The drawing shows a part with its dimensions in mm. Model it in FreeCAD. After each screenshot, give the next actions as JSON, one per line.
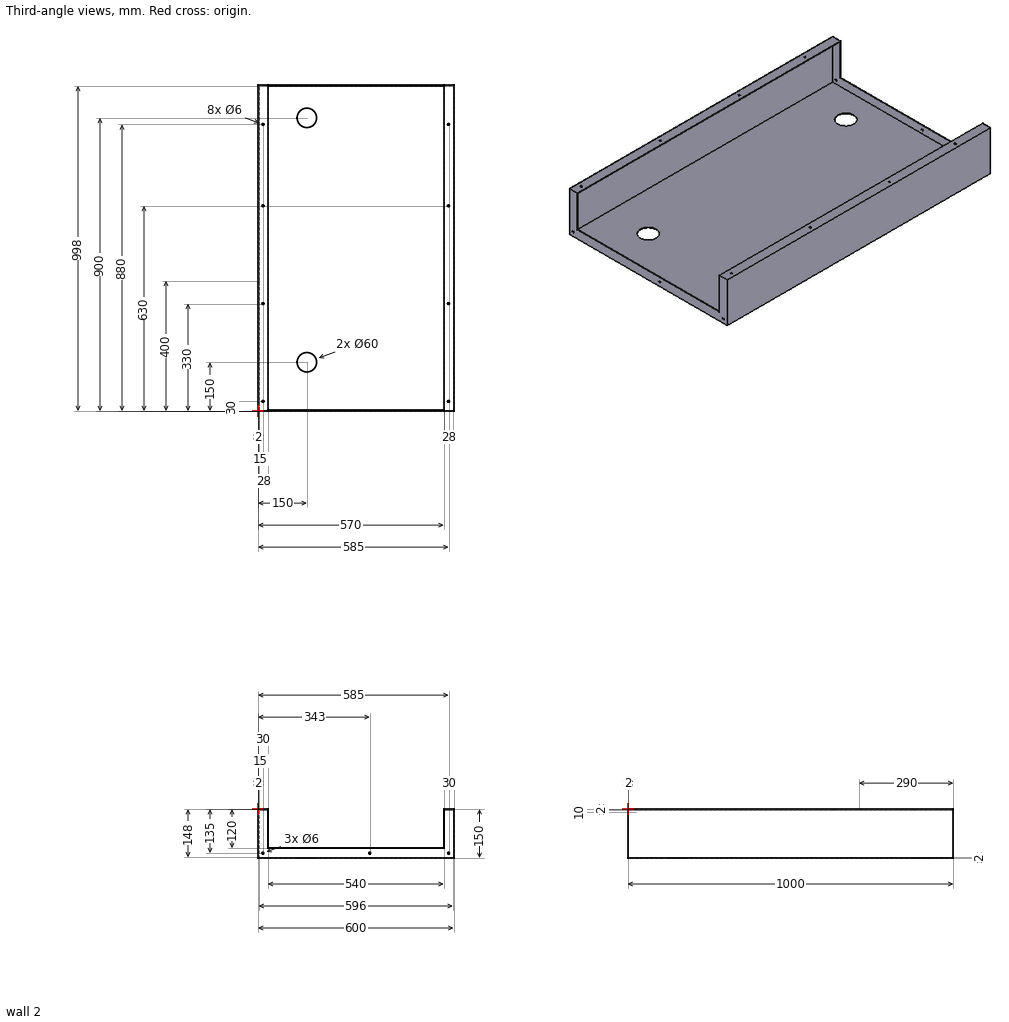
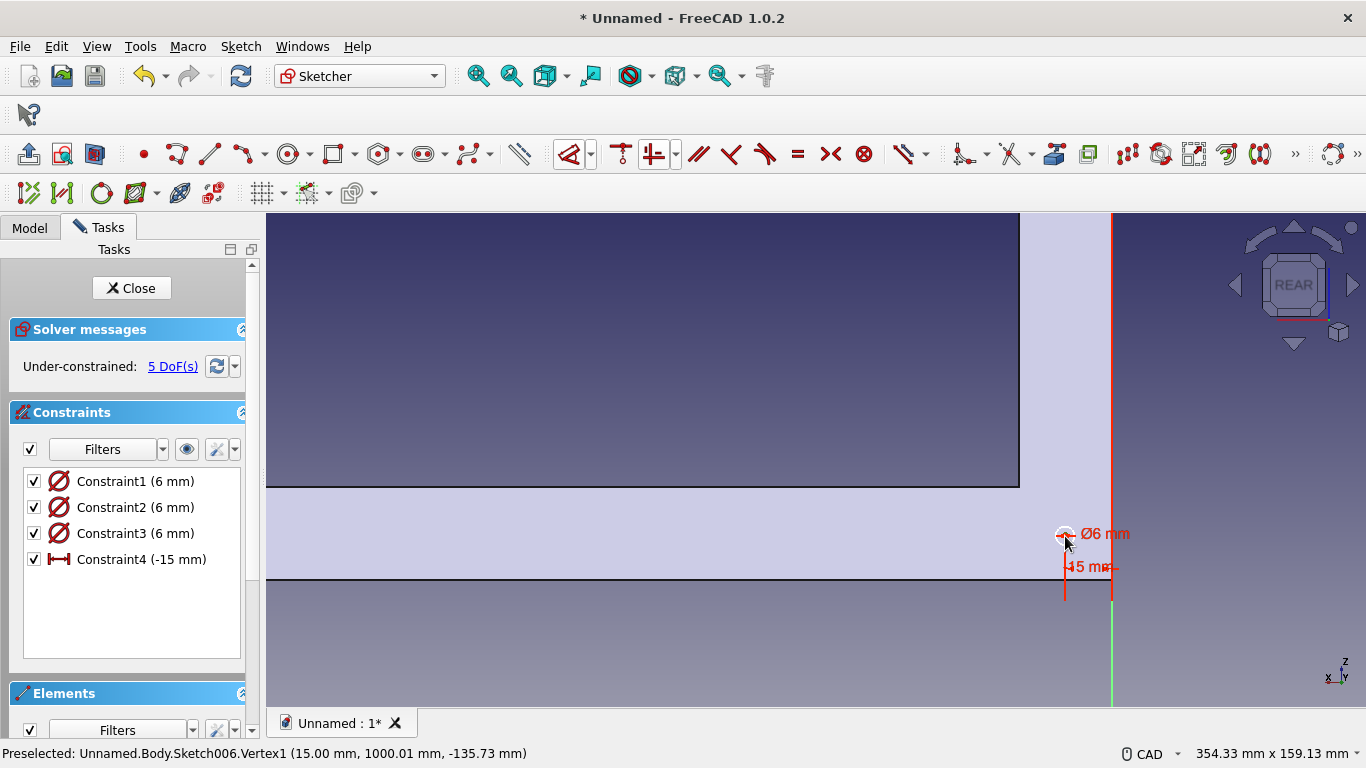
{"action": "left_click", "coordinate": [590, 154]}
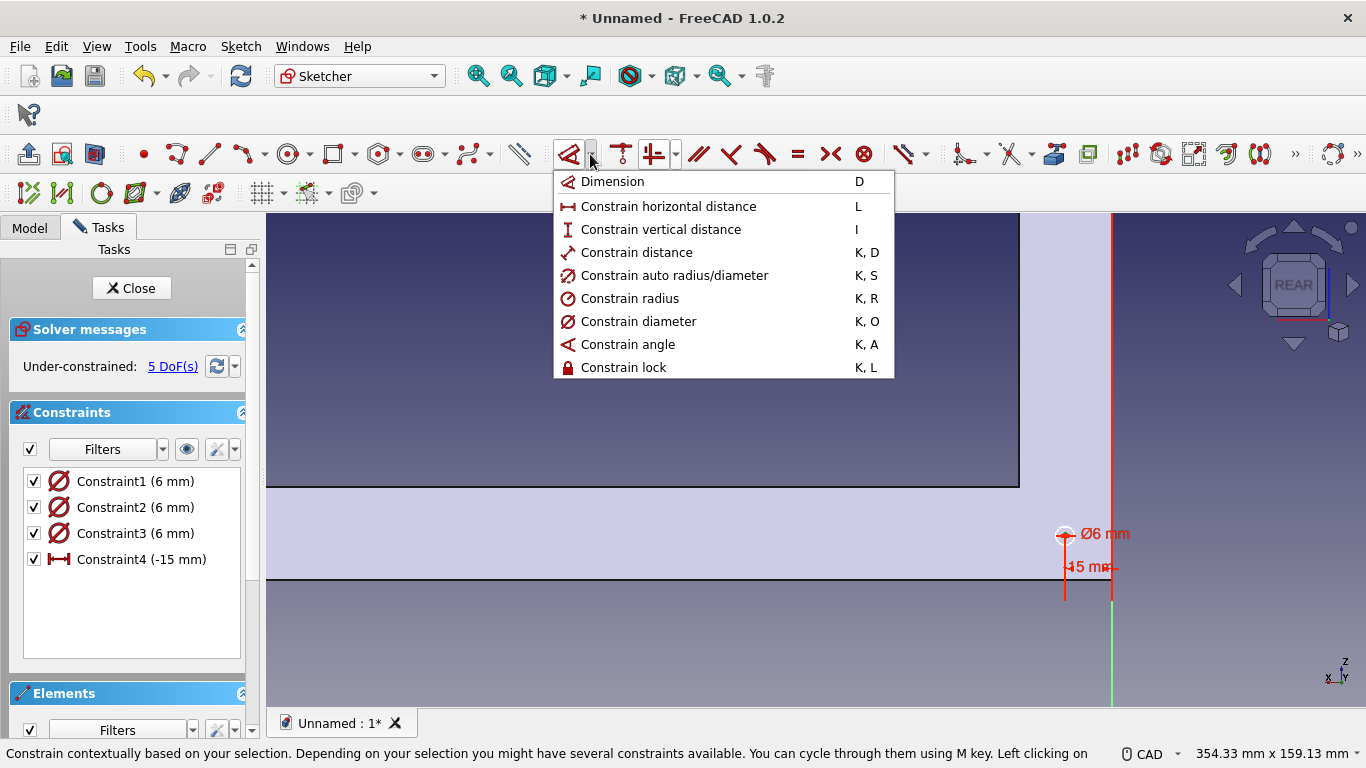
{"action": "left_click", "coordinate": [724, 230]}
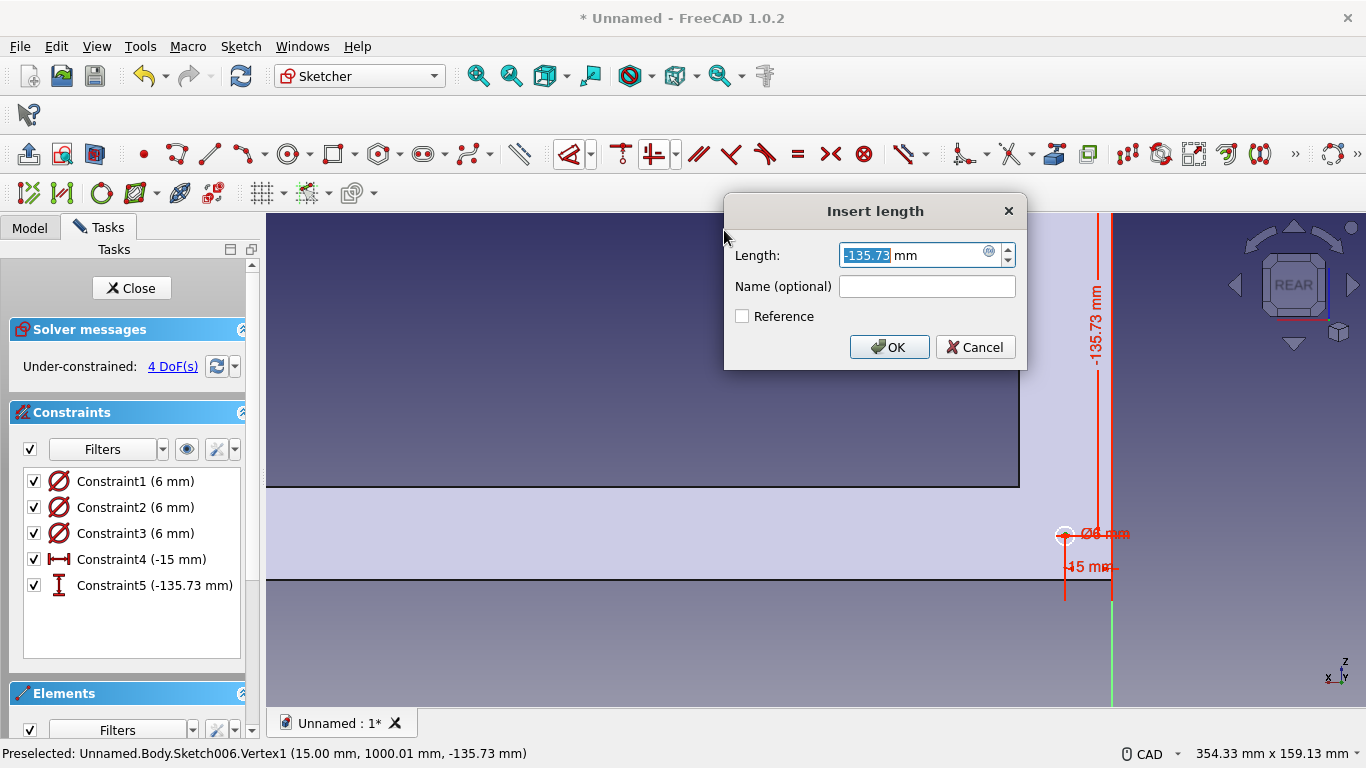
{"action": "type", "text": "-135"}
{"action": "key", "text": "Return"}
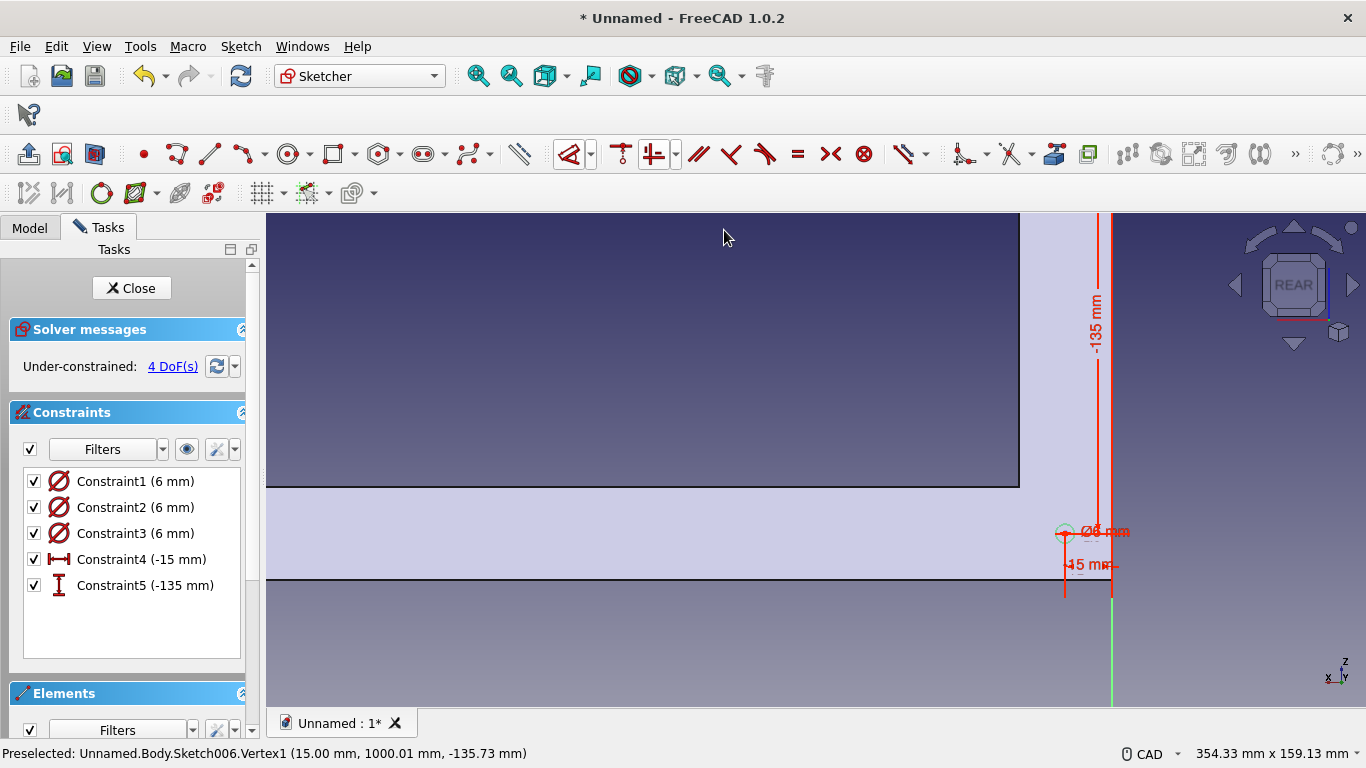
{"action": "scroll", "coordinate": [1067, 536], "scroll_direction": "down", "scroll_amount": 5}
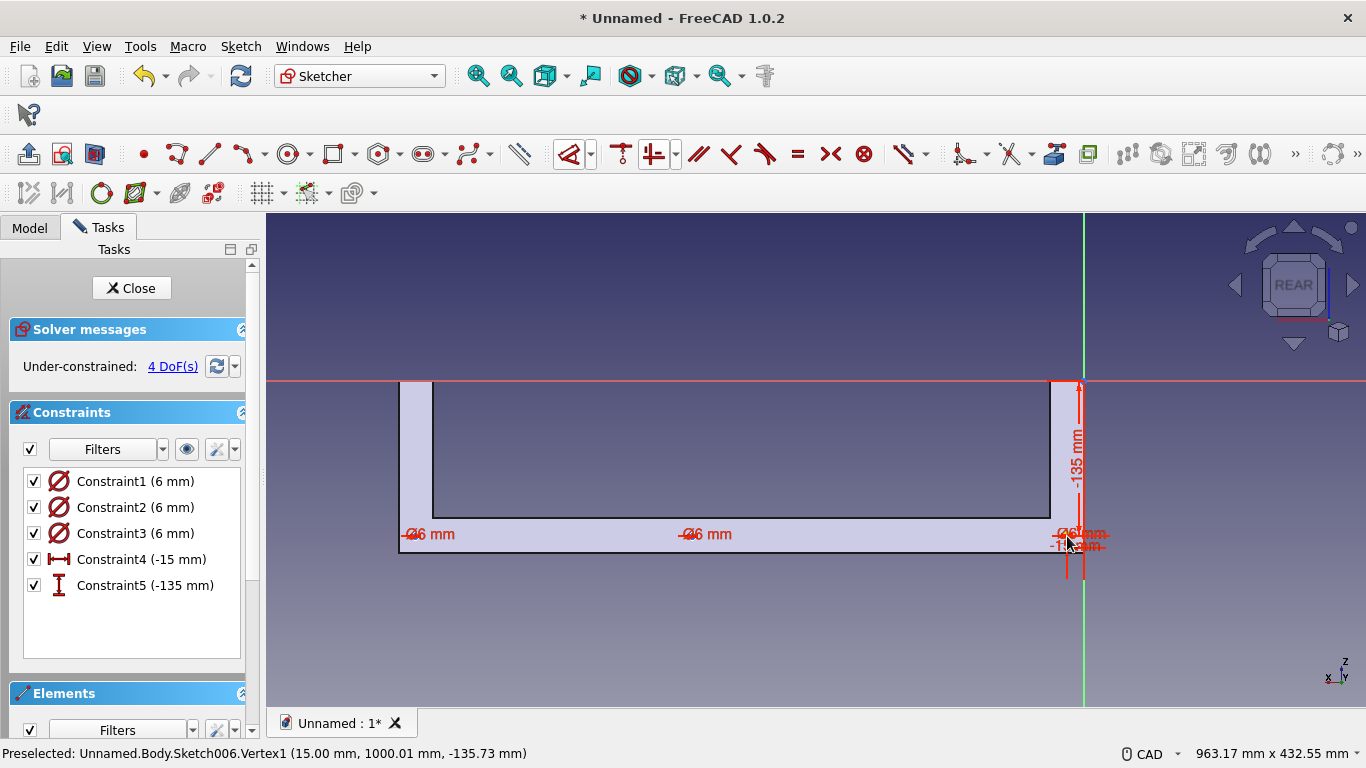
{"action": "left_click", "coordinate": [693, 536]}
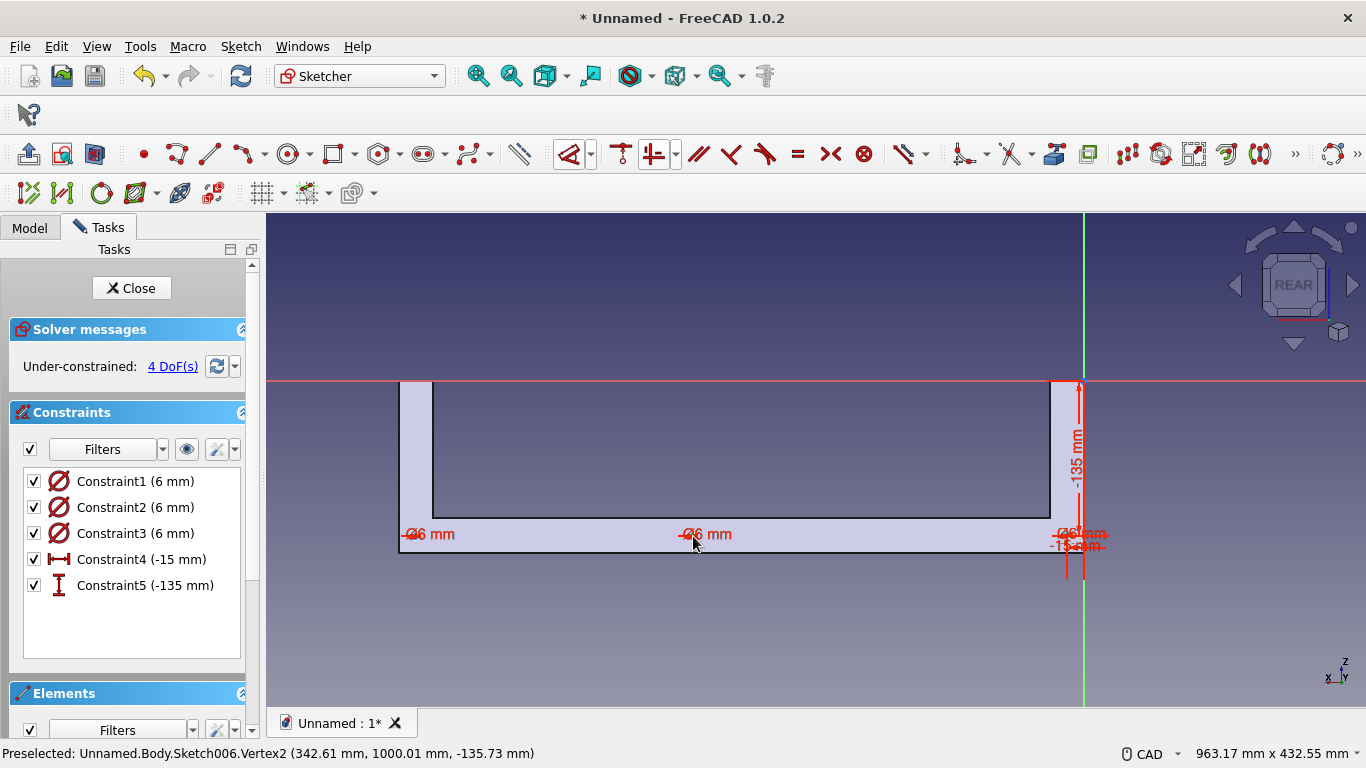
{"action": "left_click", "coordinate": [590, 154]}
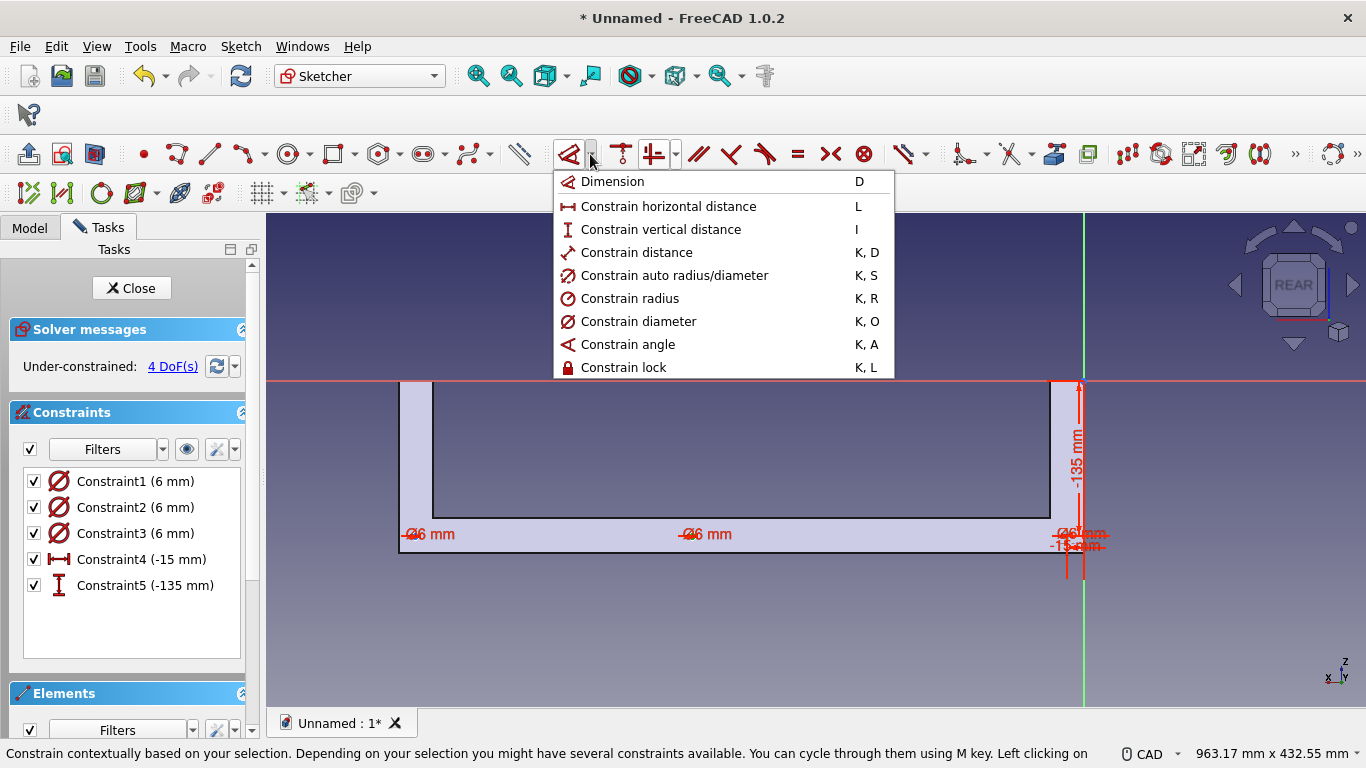
{"action": "left_click", "coordinate": [724, 206]}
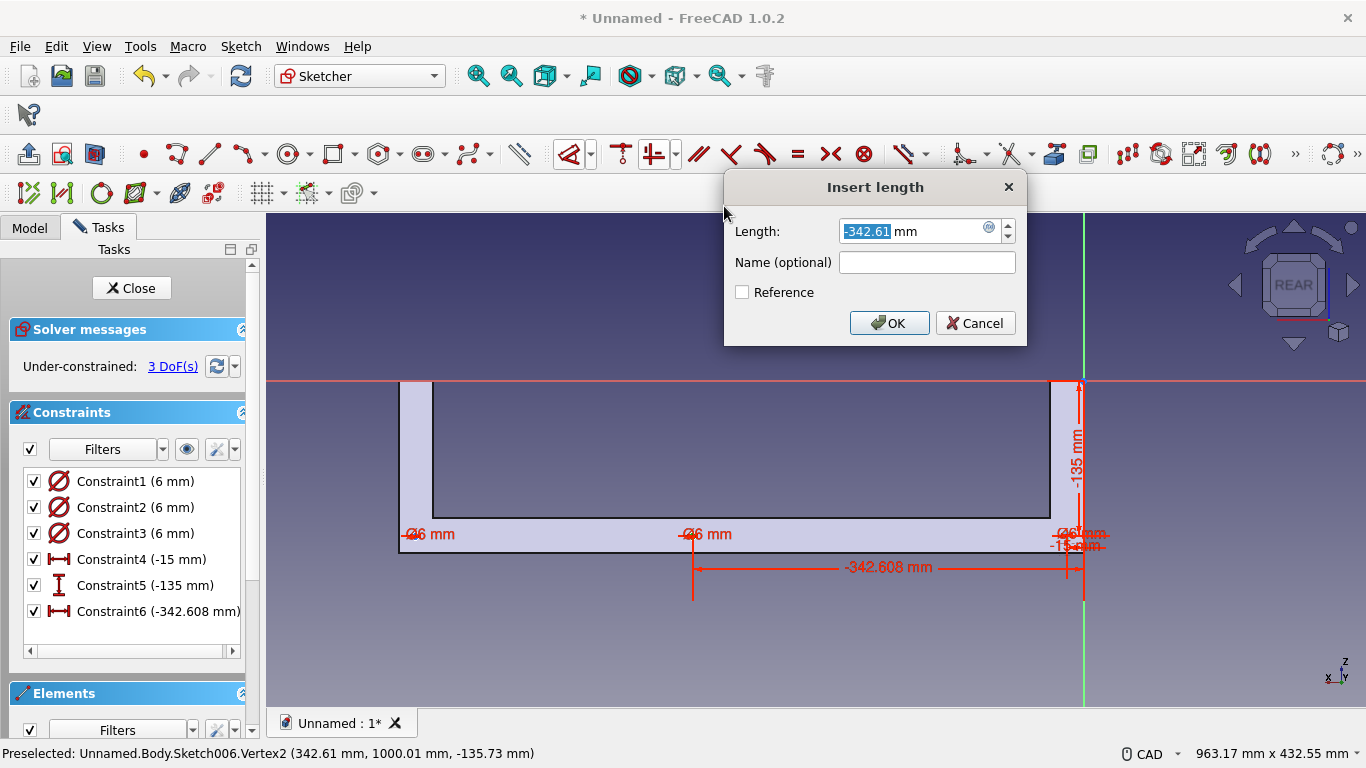
{"action": "type", "text": "-343"}
{"action": "key", "text": "Return"}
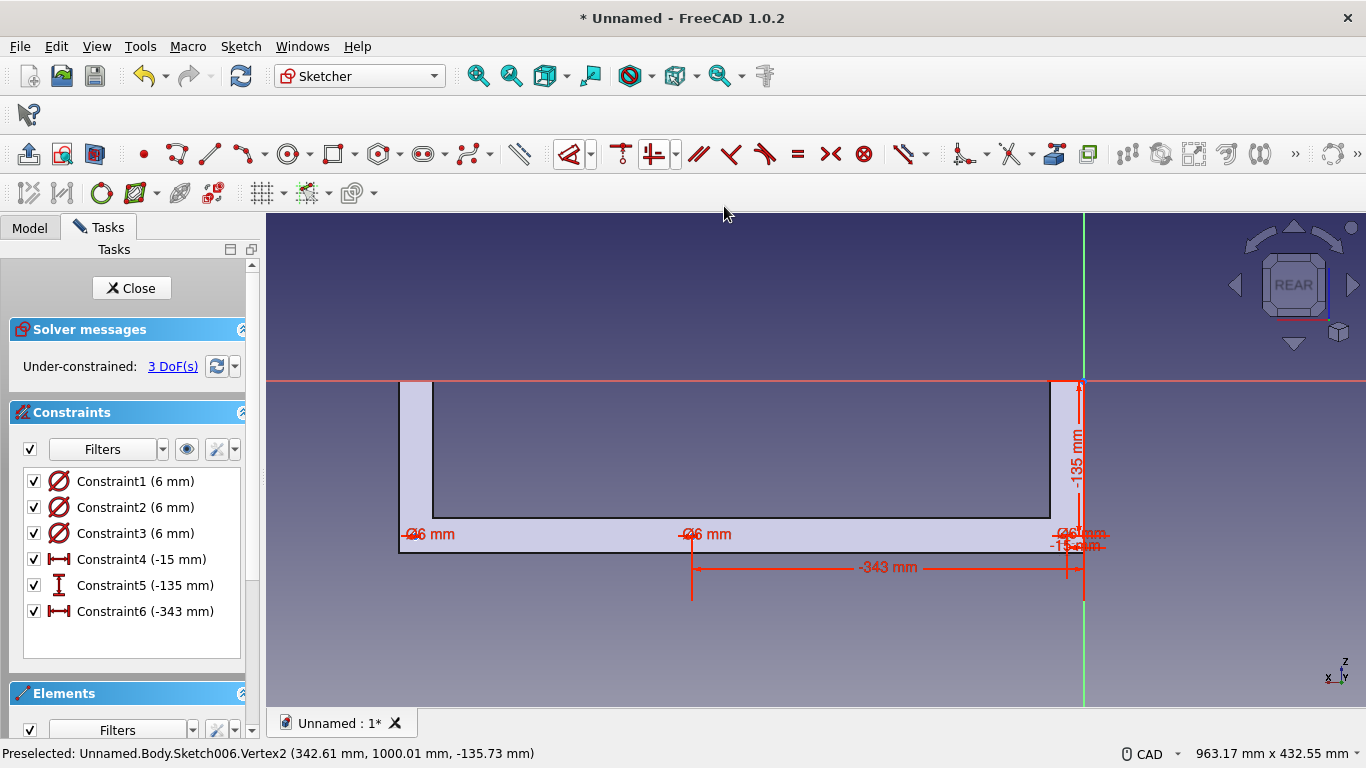
{"action": "left_click", "coordinate": [692, 536]}